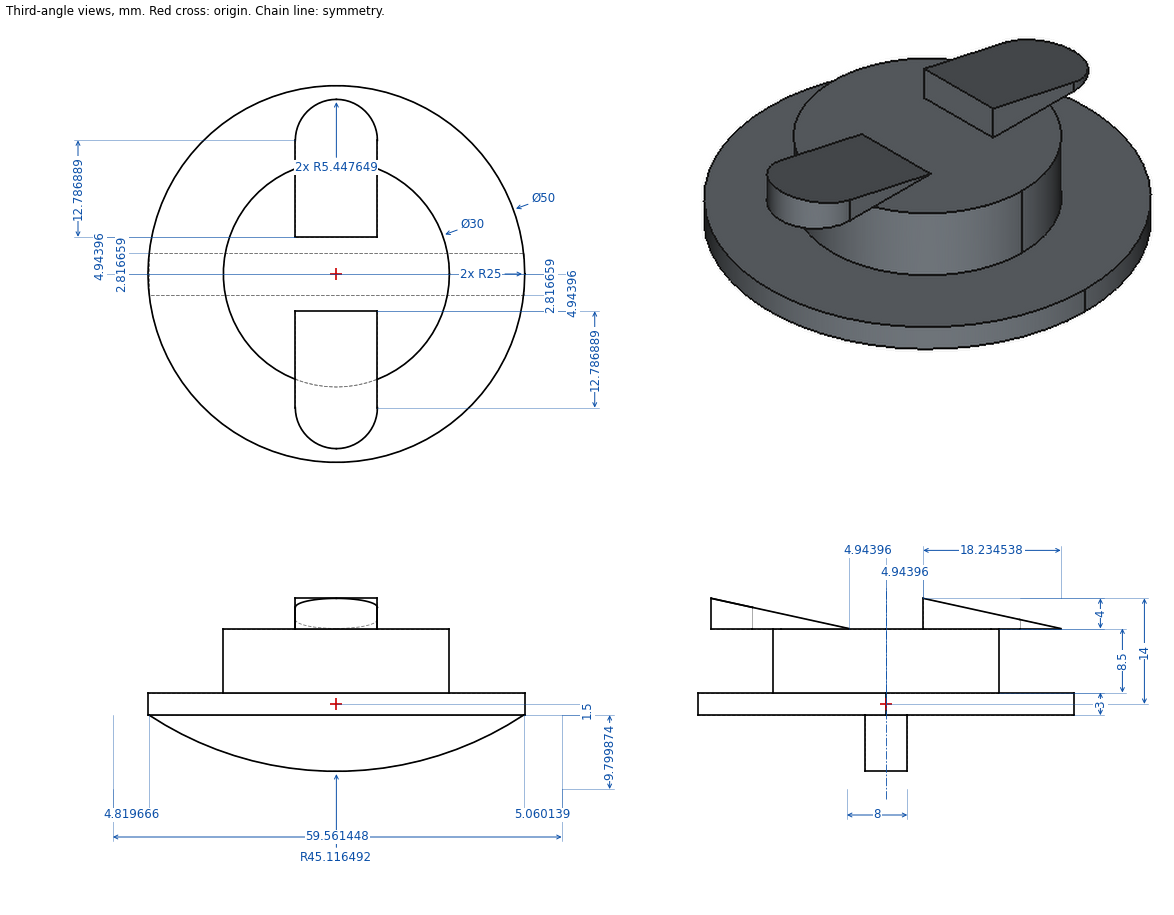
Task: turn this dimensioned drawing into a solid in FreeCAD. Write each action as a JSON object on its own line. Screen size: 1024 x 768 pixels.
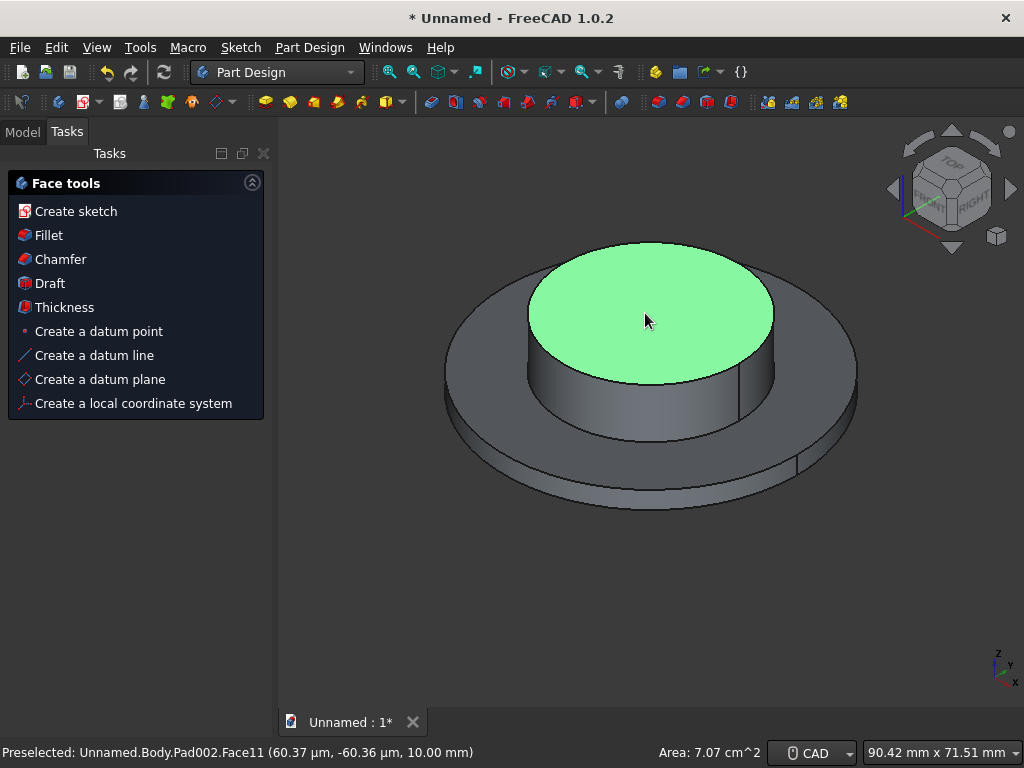
{"action": "left_click", "coordinate": [84, 102]}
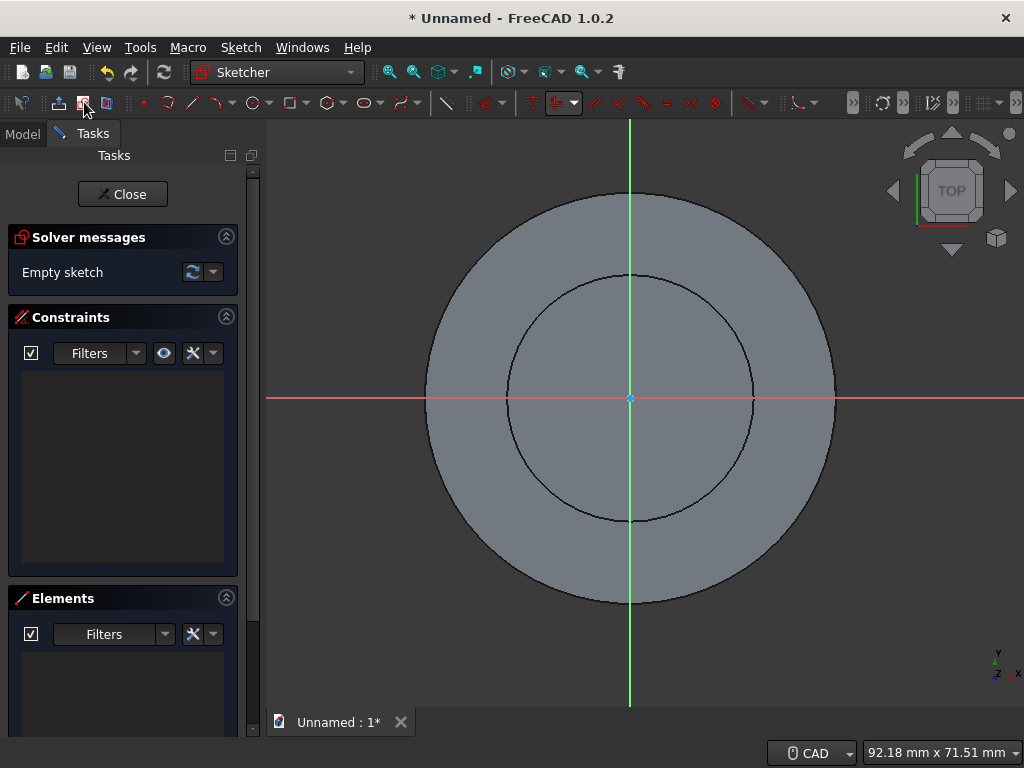
{"action": "left_click", "coordinate": [168, 104]}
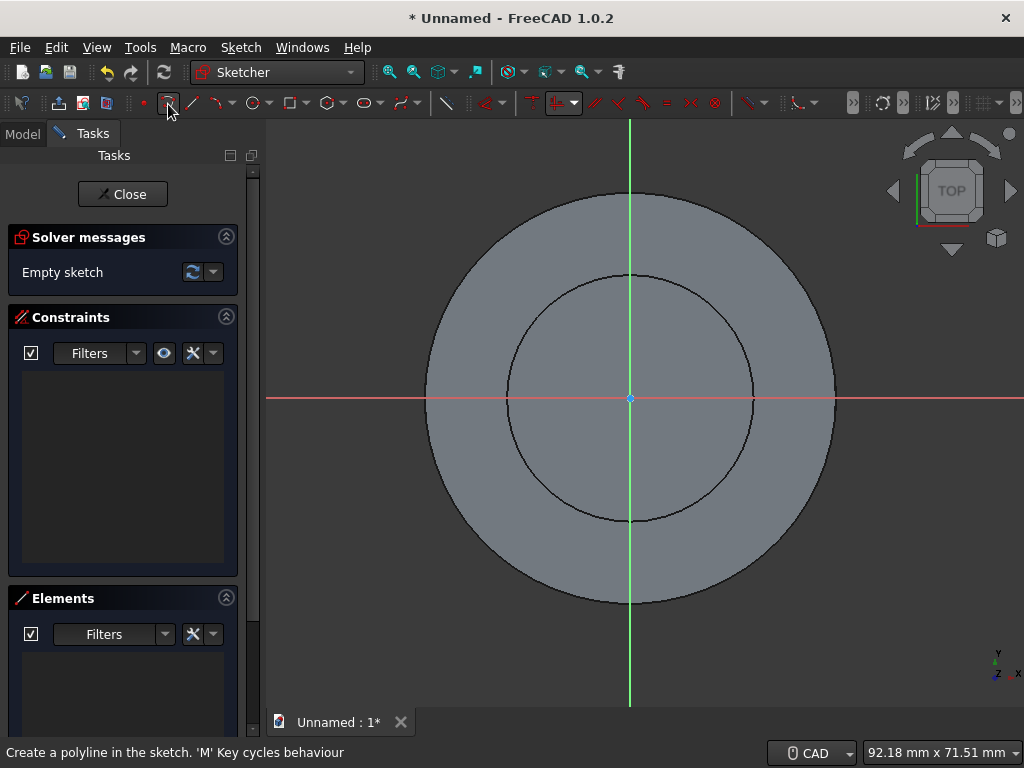
{"action": "left_click", "coordinate": [586, 253]}
{"action": "left_click", "coordinate": [586, 358]}
{"action": "left_click", "coordinate": [675, 358]}
{"action": "left_click", "coordinate": [675, 253]}
{"action": "right_click", "coordinate": [675, 253]}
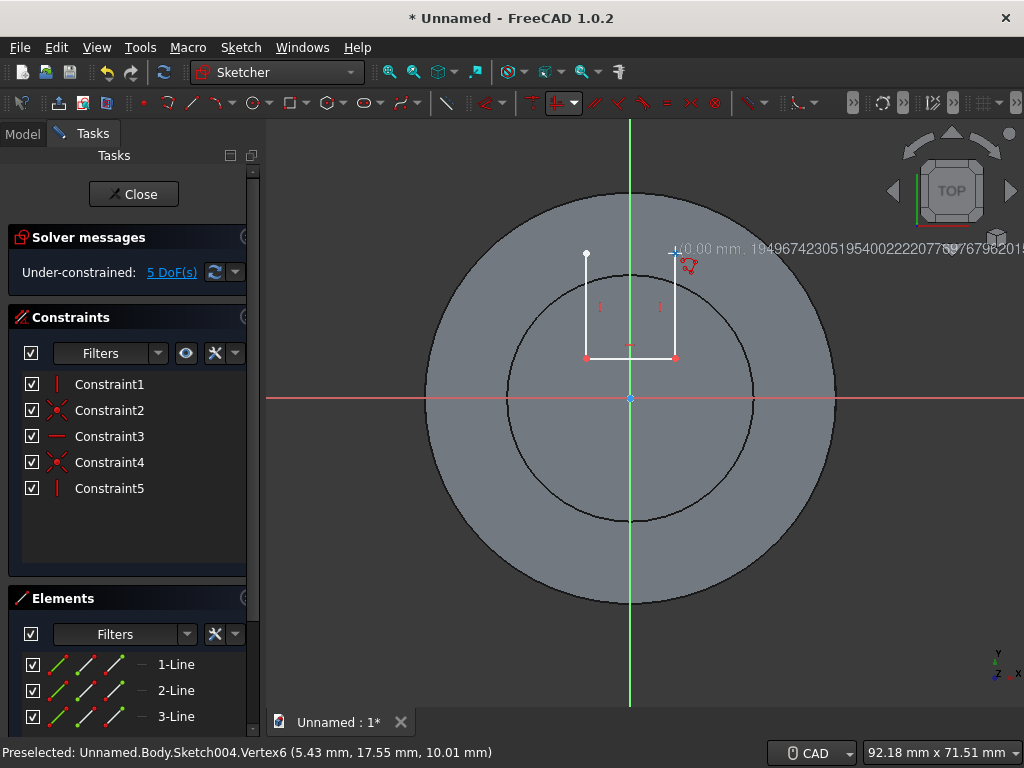
{"action": "left_click", "coordinate": [216, 104]}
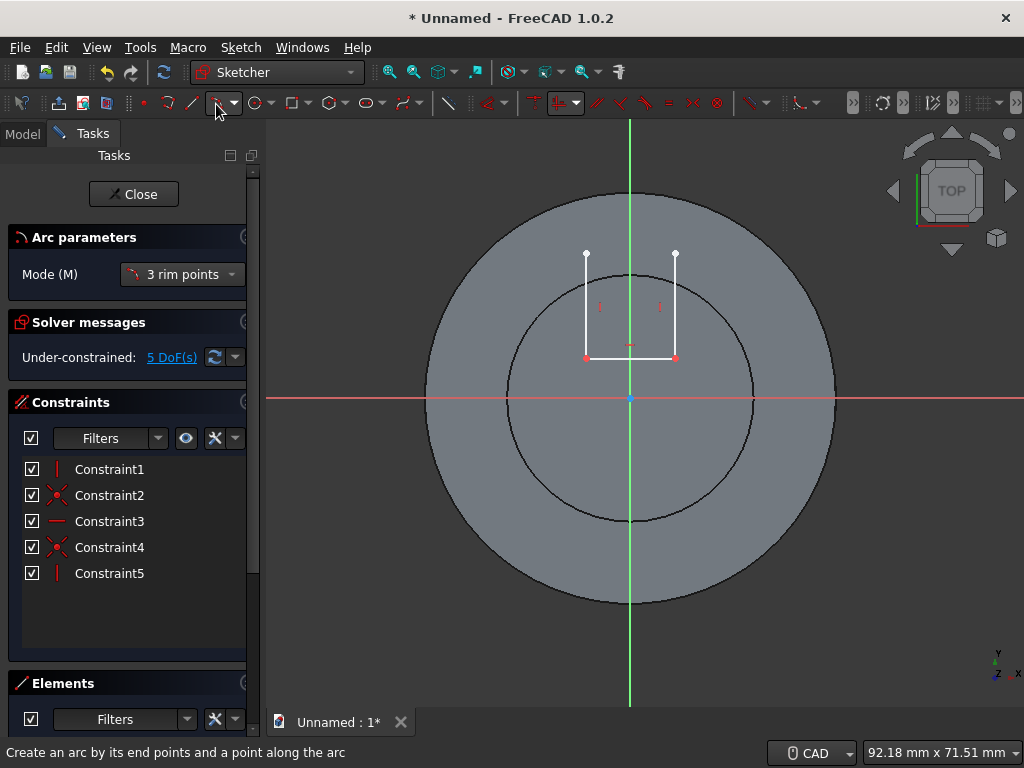
{"action": "left_click", "coordinate": [675, 254]}
{"action": "left_click", "coordinate": [586, 254]}
{"action": "left_click", "coordinate": [657, 216]}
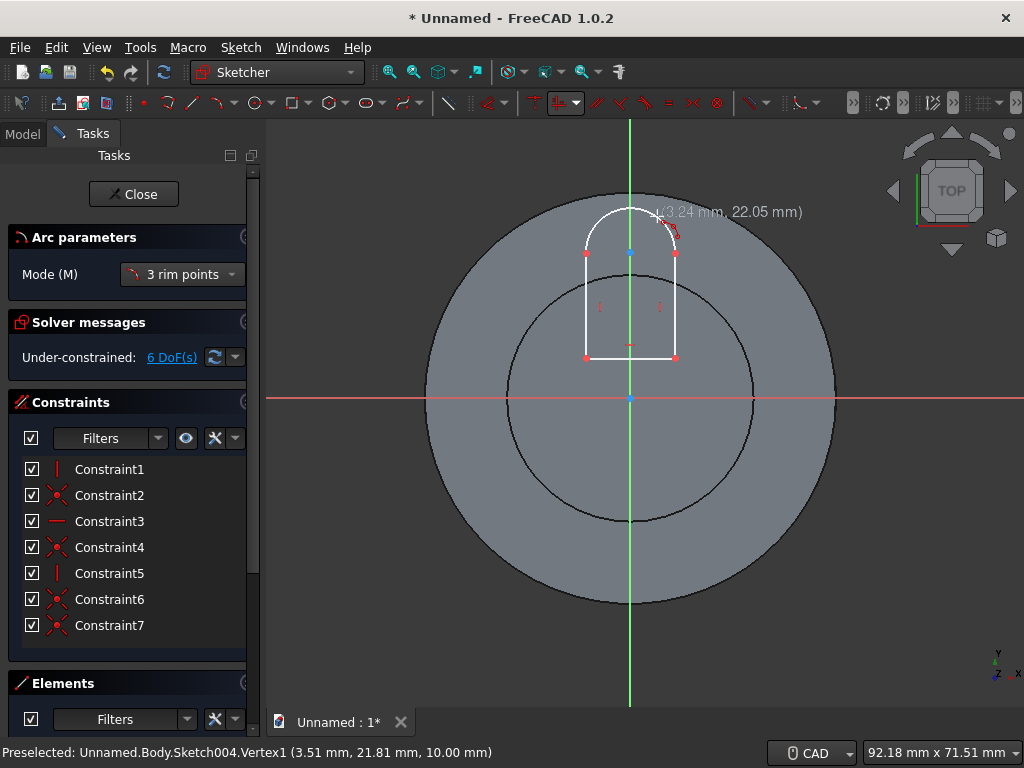
{"action": "left_click", "coordinate": [168, 104]}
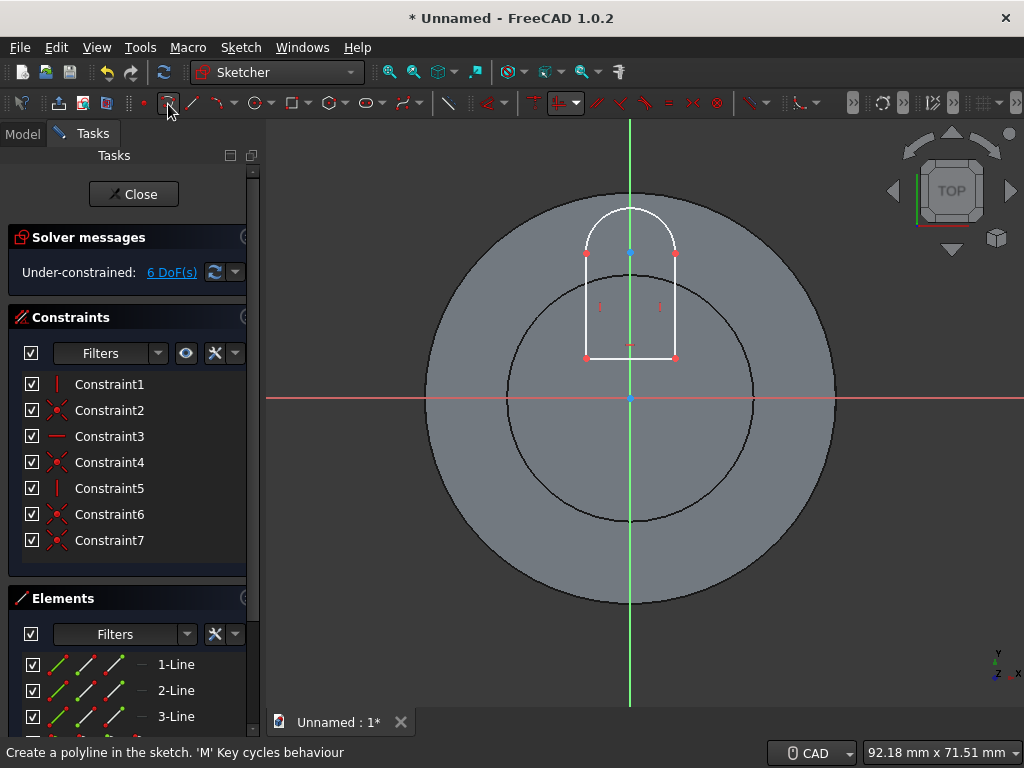
{"action": "left_click", "coordinate": [675, 544]}
{"action": "left_click", "coordinate": [675, 439]}
{"action": "left_click", "coordinate": [586, 439]}
{"action": "left_click", "coordinate": [586, 544]}
{"action": "right_click", "coordinate": [586, 544]}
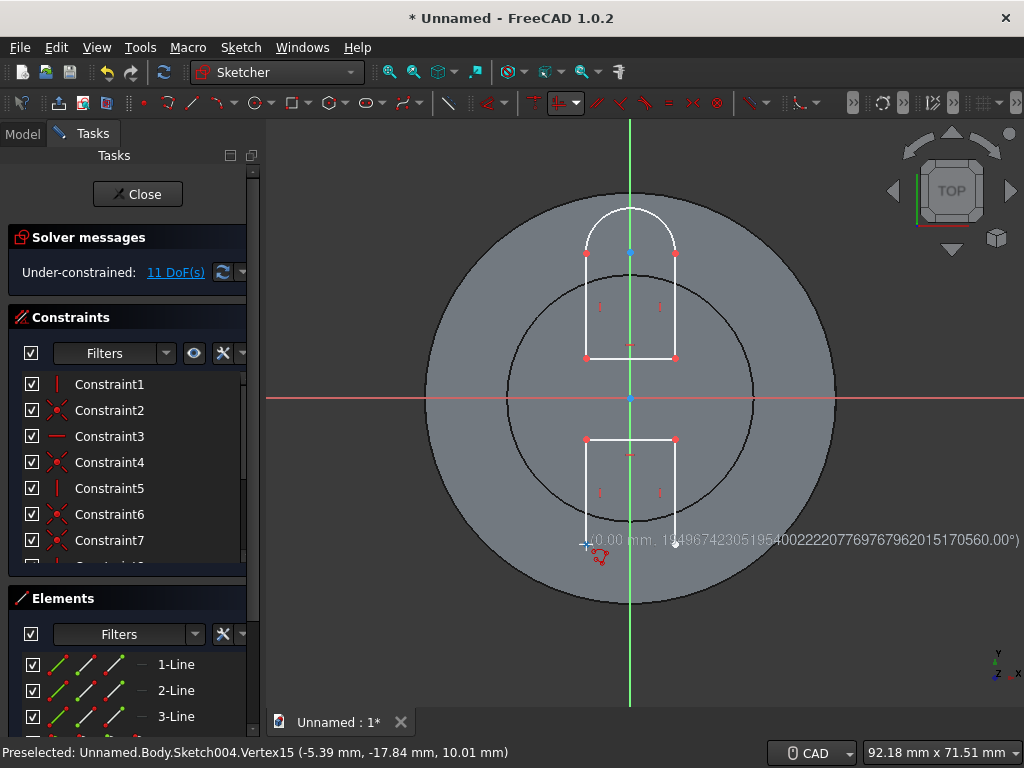
{"action": "left_click", "coordinate": [218, 104]}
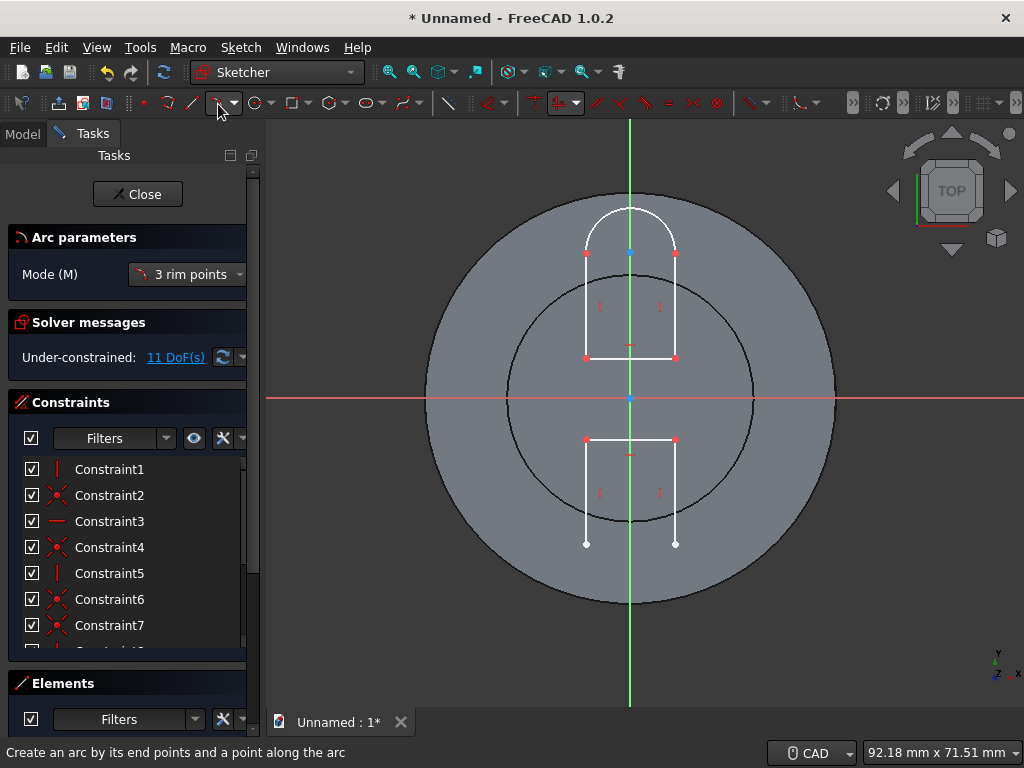
{"action": "left_click", "coordinate": [586, 545]}
{"action": "left_click", "coordinate": [675, 545]}
{"action": "left_click", "coordinate": [604, 580]}
{"action": "key", "text": "Escape"}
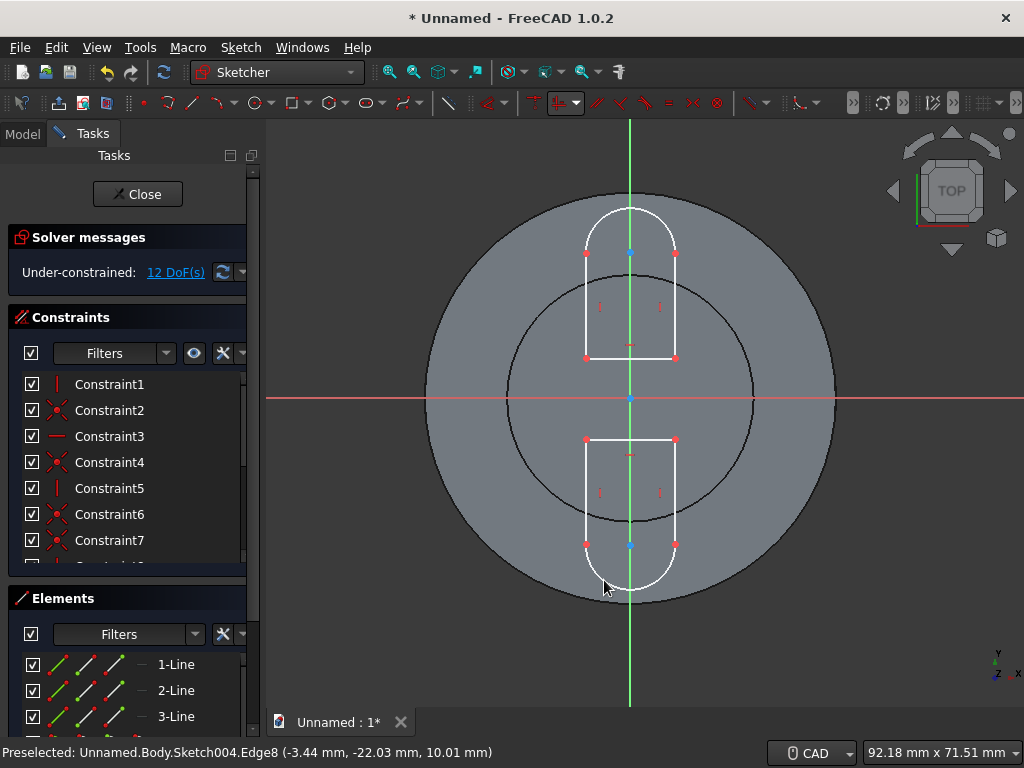
{"action": "left_click", "coordinate": [586, 286]}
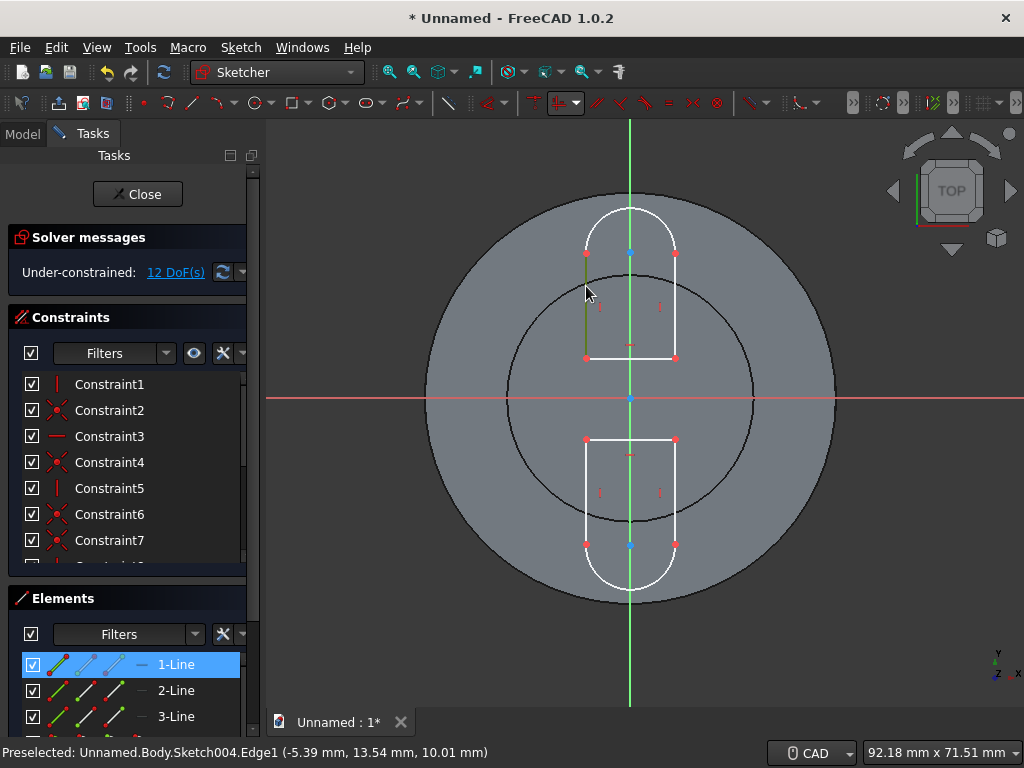
{"action": "left_click", "coordinate": [657, 217]}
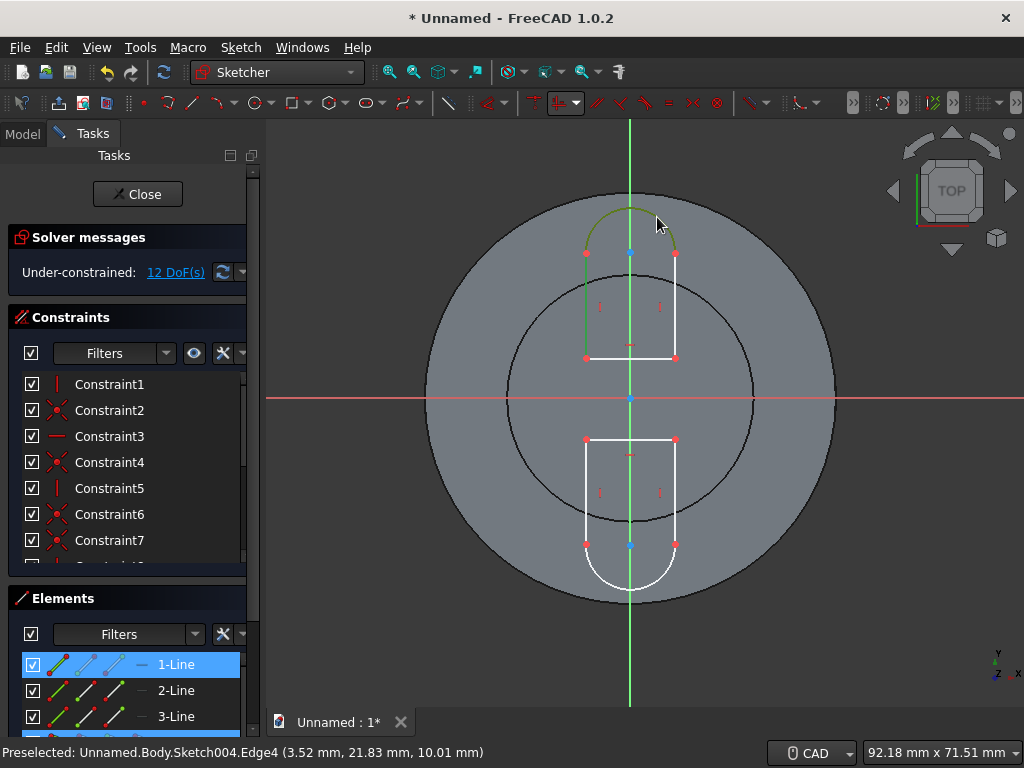
{"action": "left_click", "coordinate": [646, 104]}